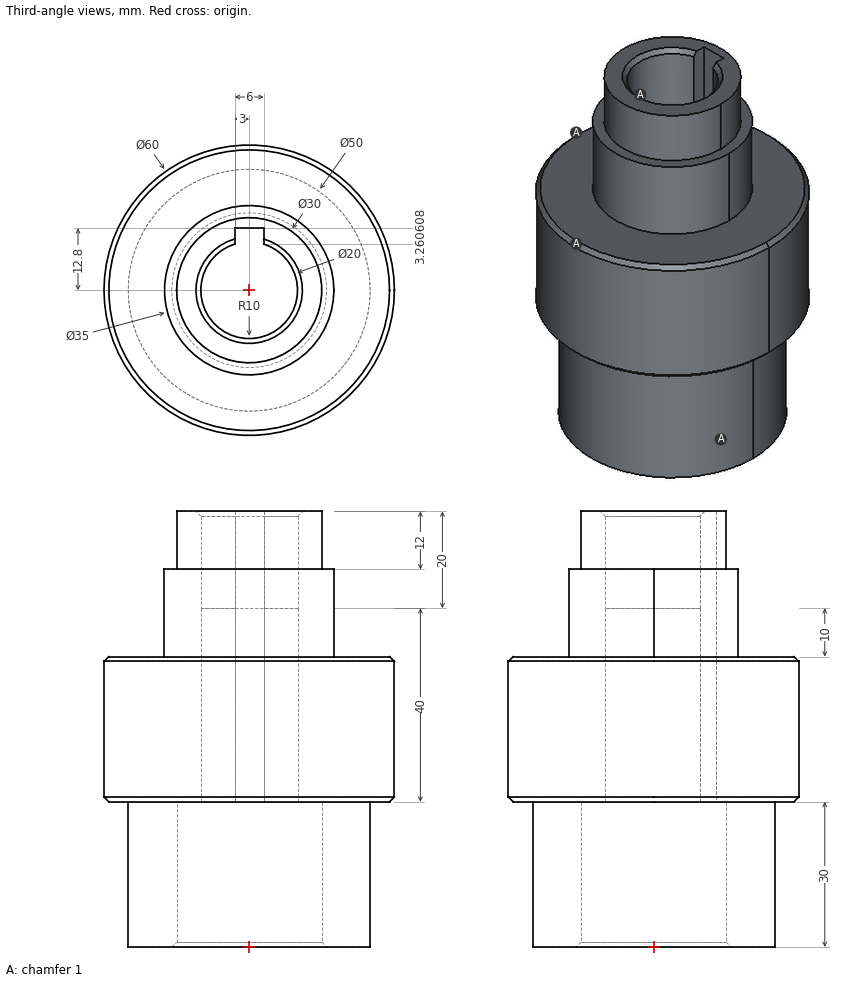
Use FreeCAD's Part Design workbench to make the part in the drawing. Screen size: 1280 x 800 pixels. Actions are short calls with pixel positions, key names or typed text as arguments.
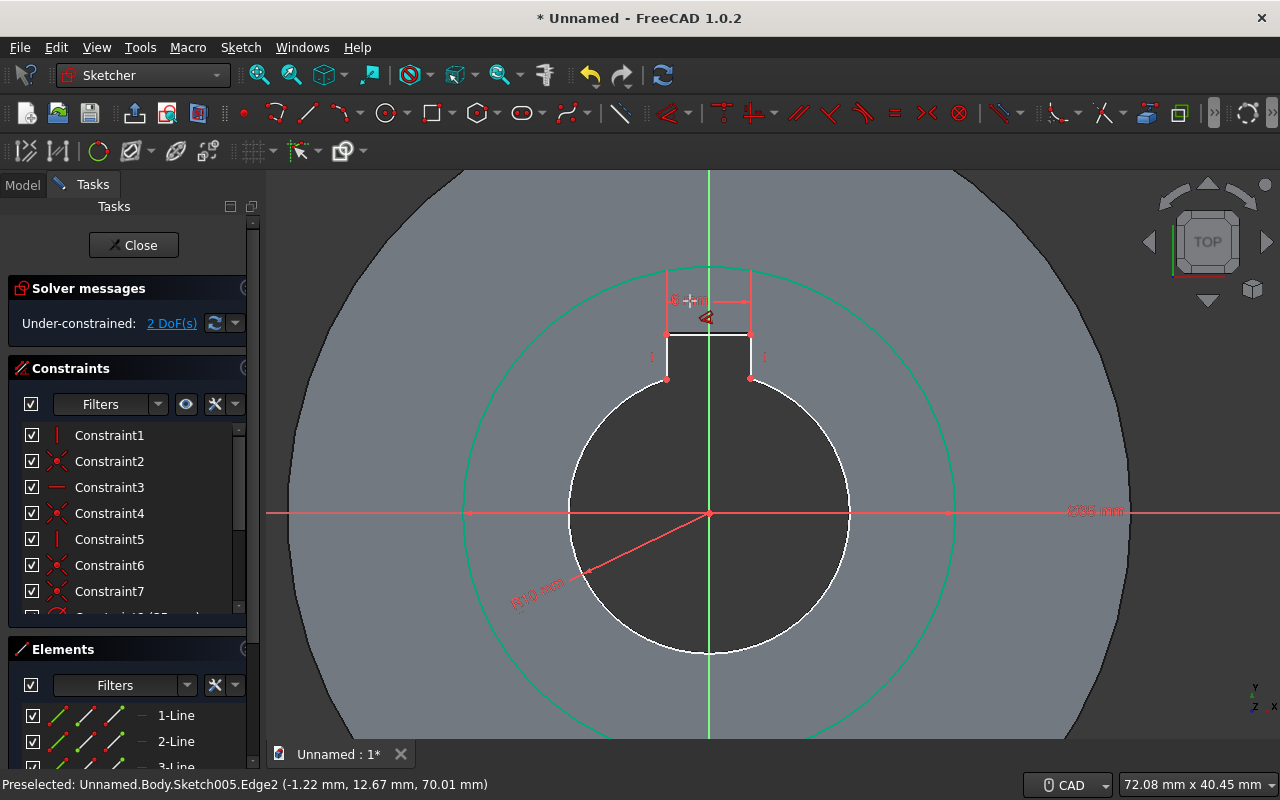
click(667, 379)
click(688, 547)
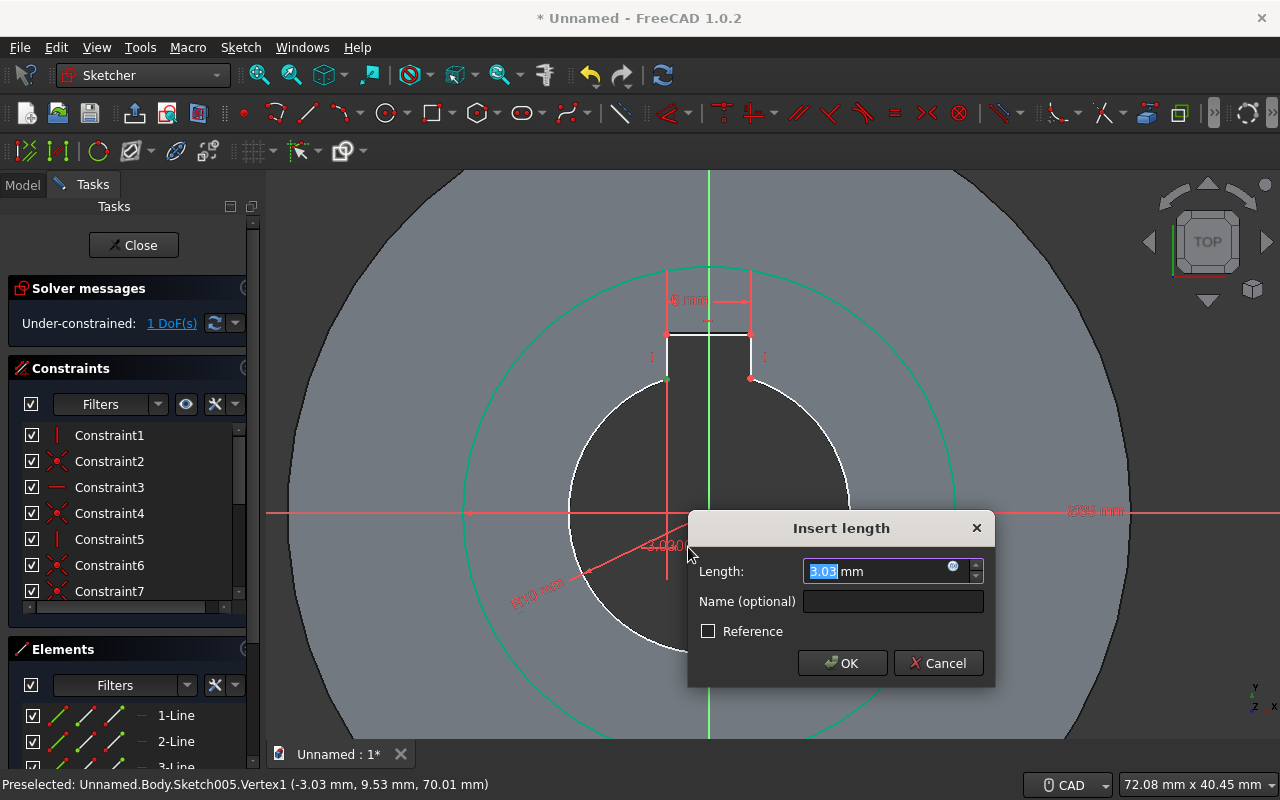
text(3)
key(Return)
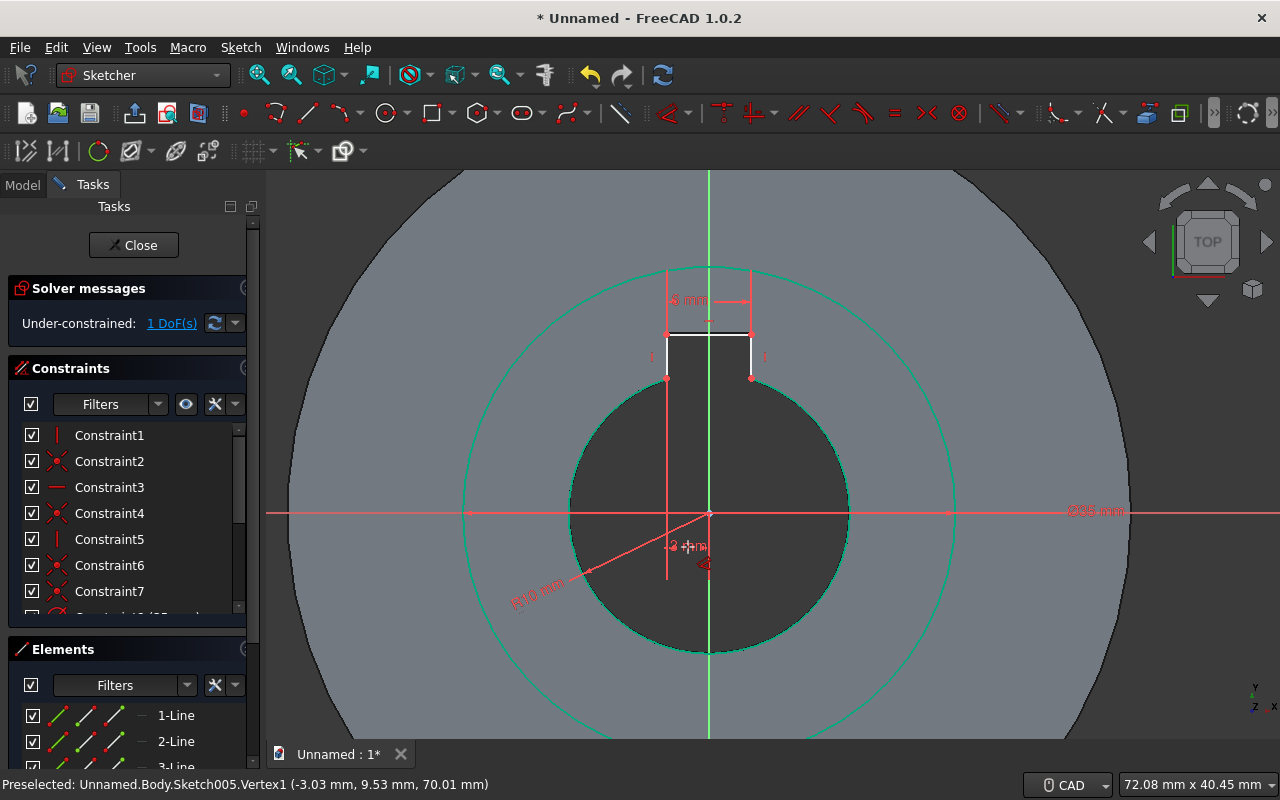
click(667, 335)
click(633, 424)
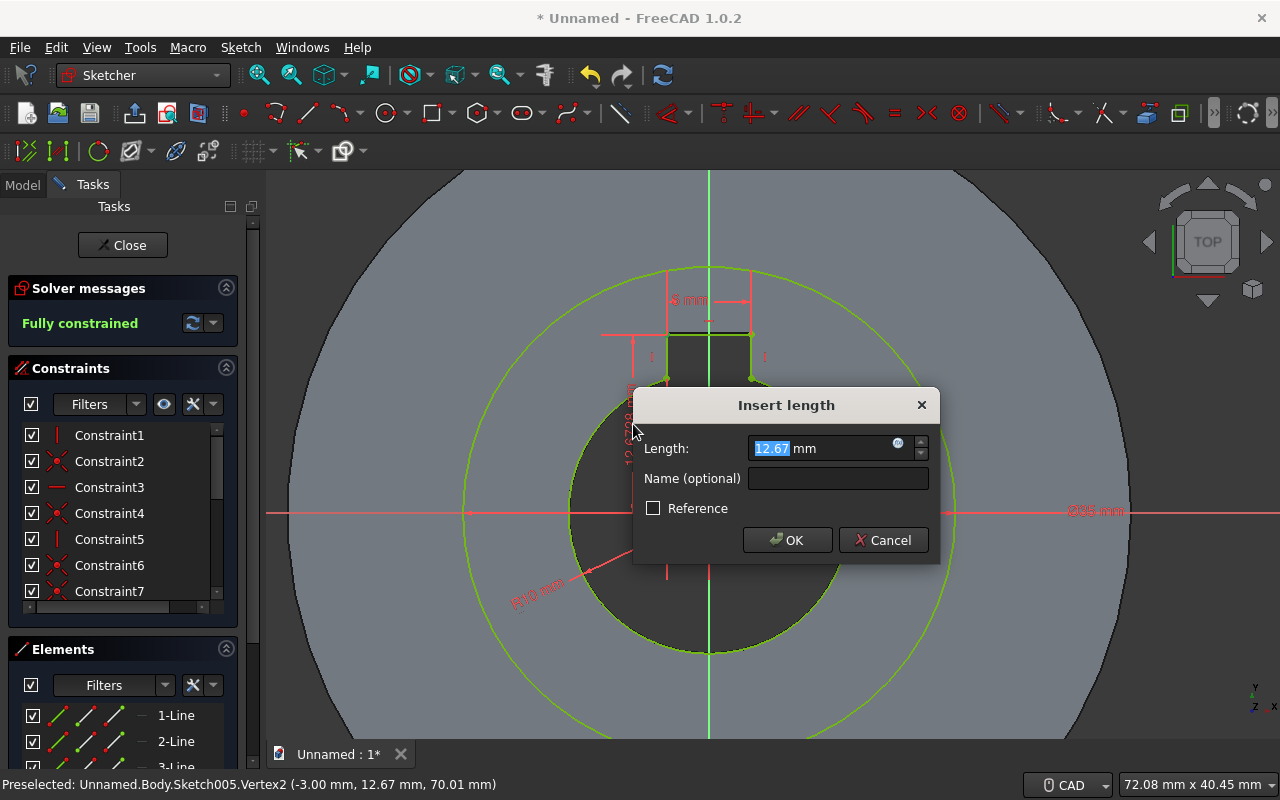
text(12.8)
key(Return)
key(Escape)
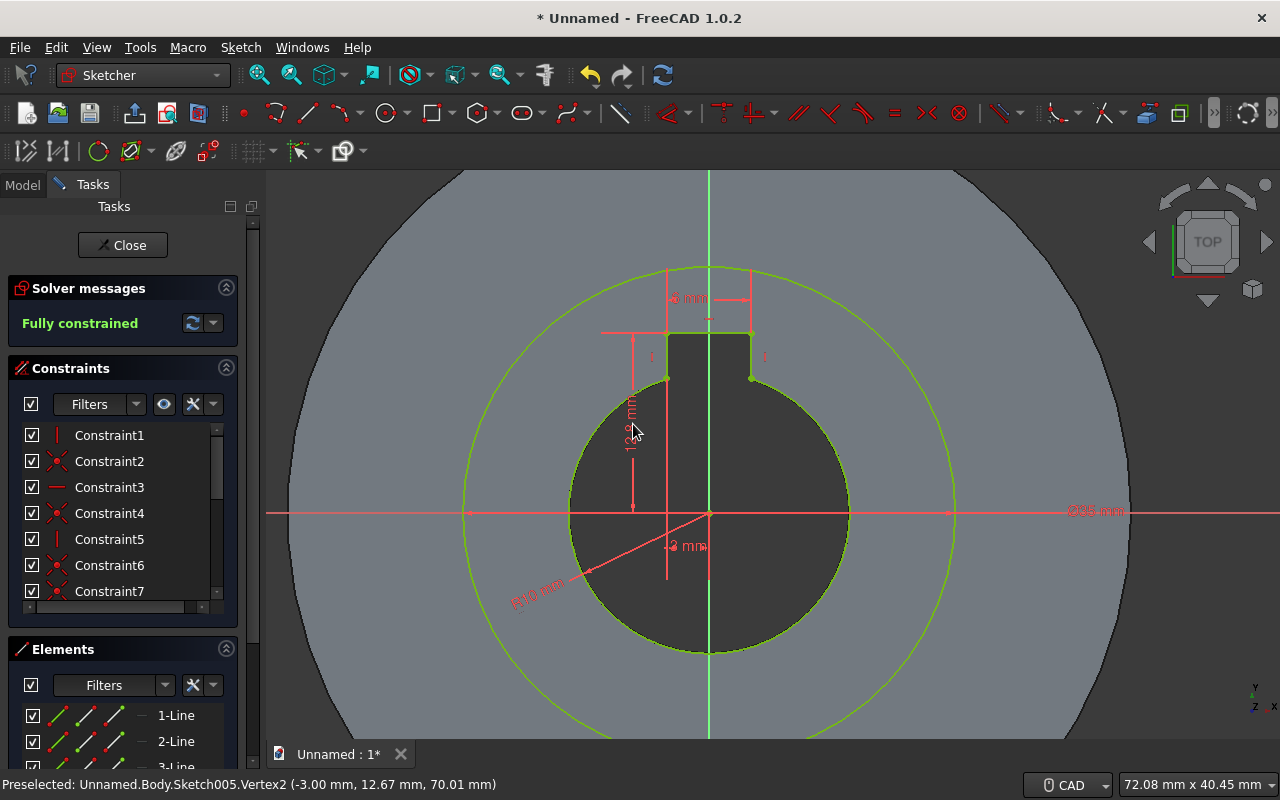
click(123, 245)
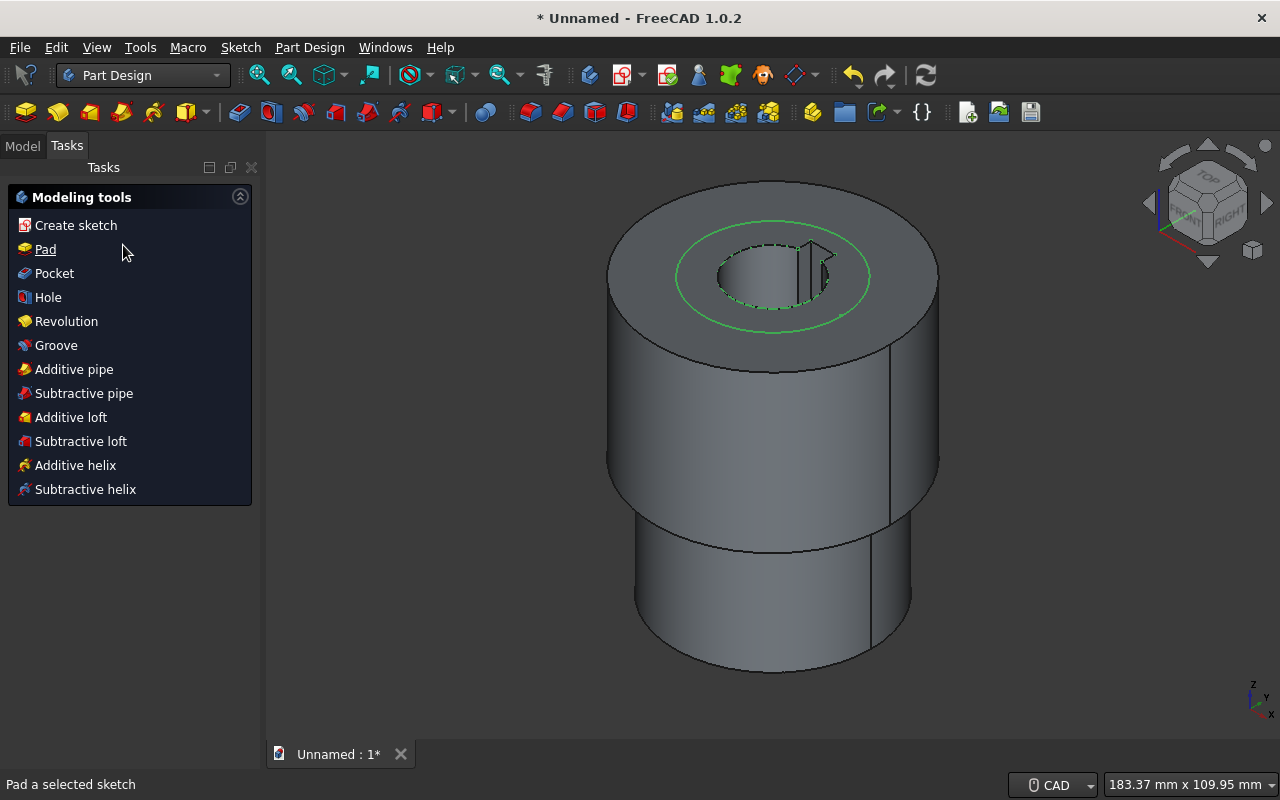
click(26, 112)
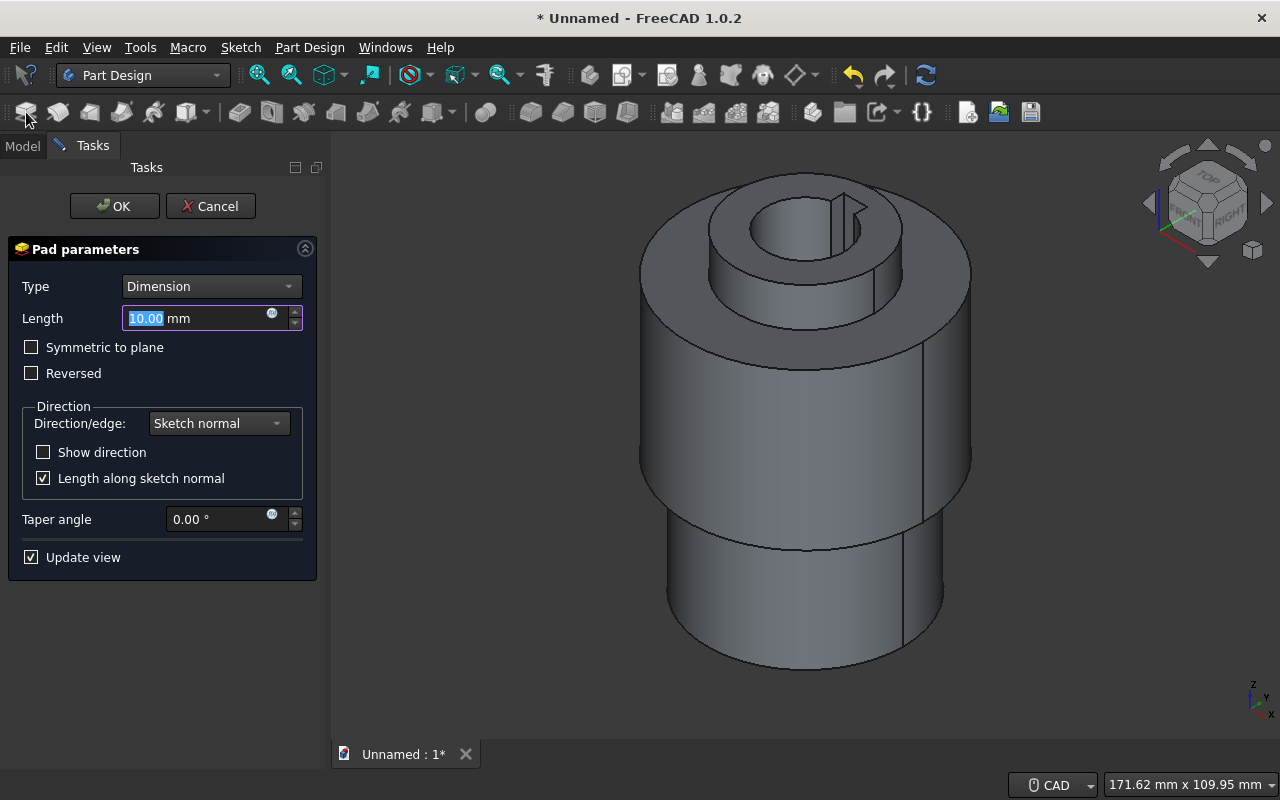
text(20)
key(Tab)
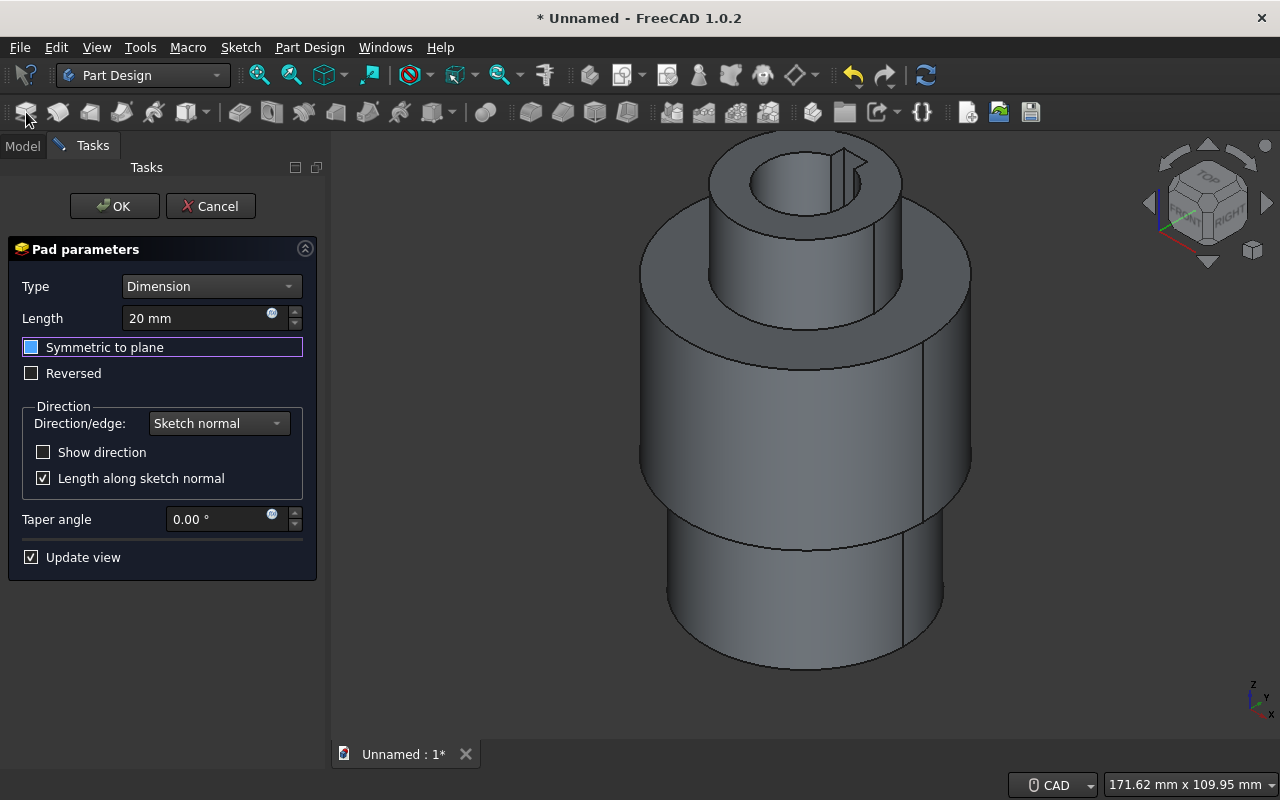
click(115, 206)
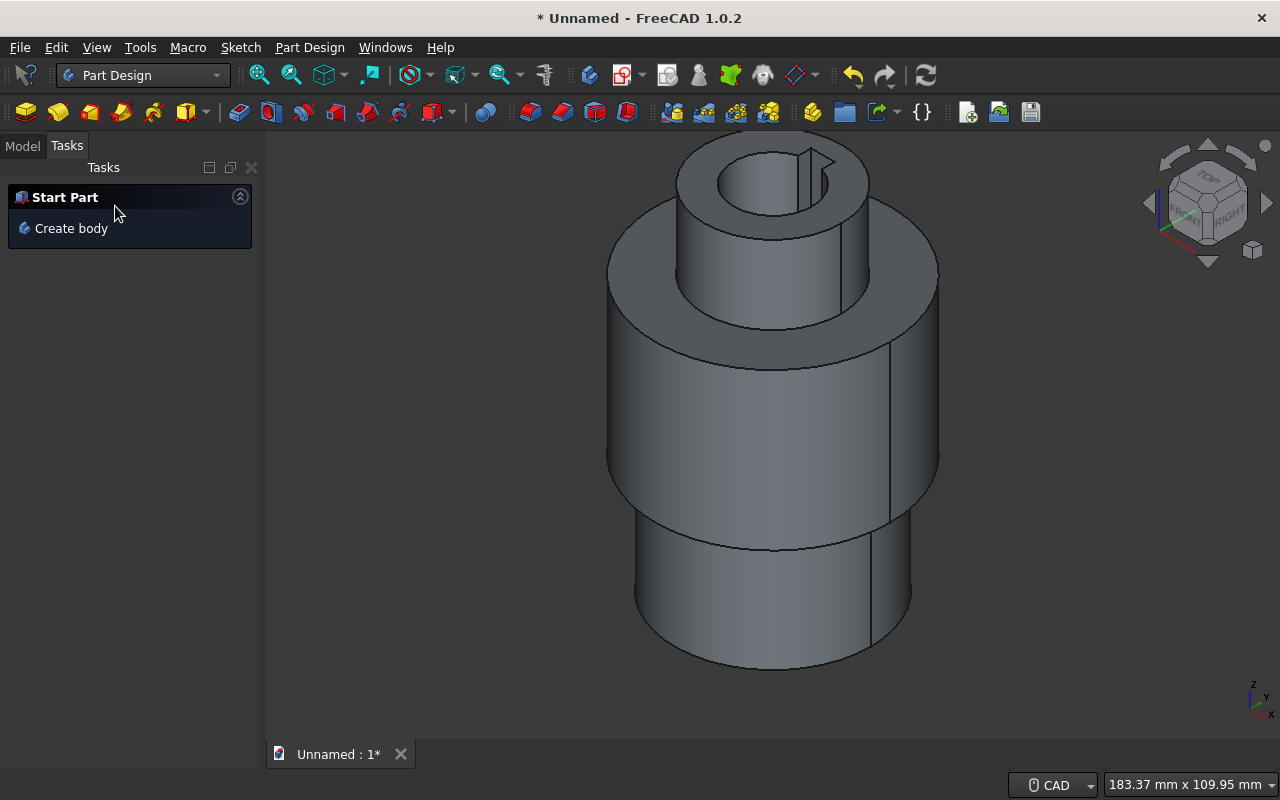
click(260, 76)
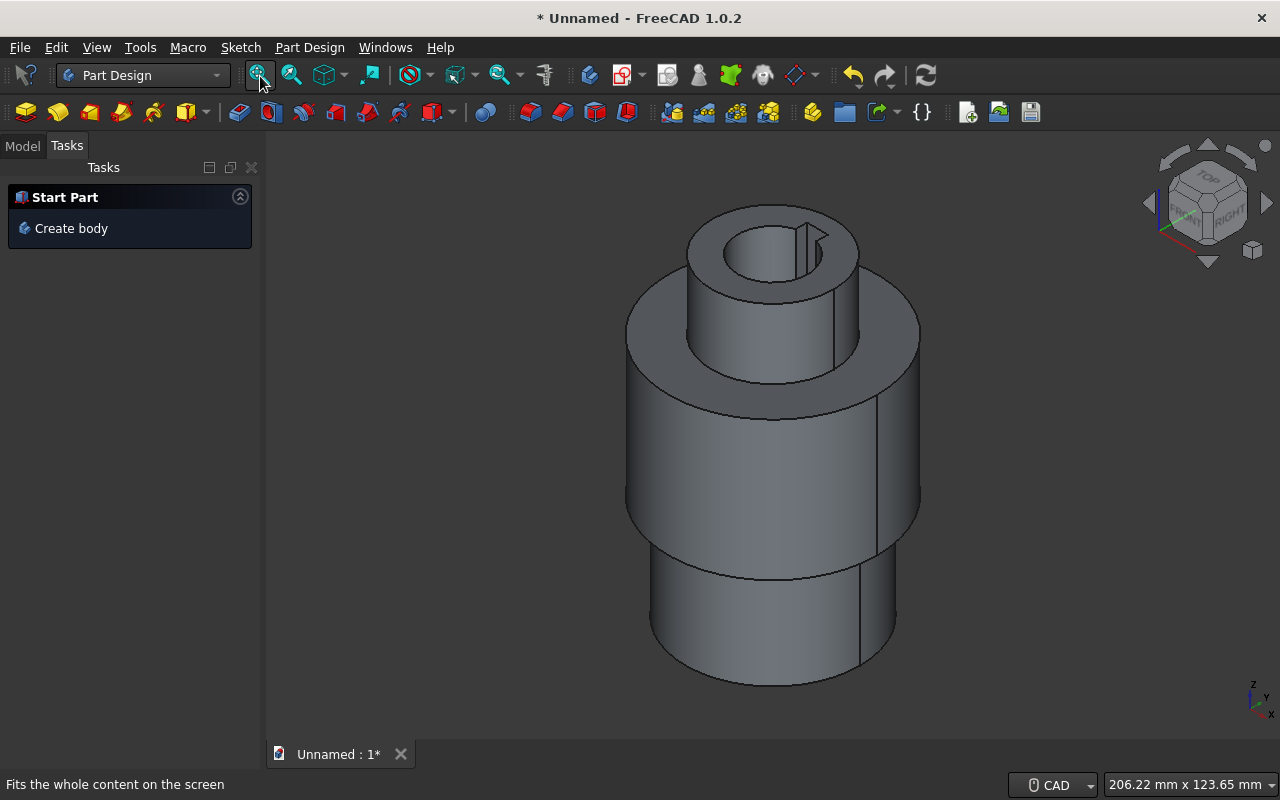
click(23, 145)